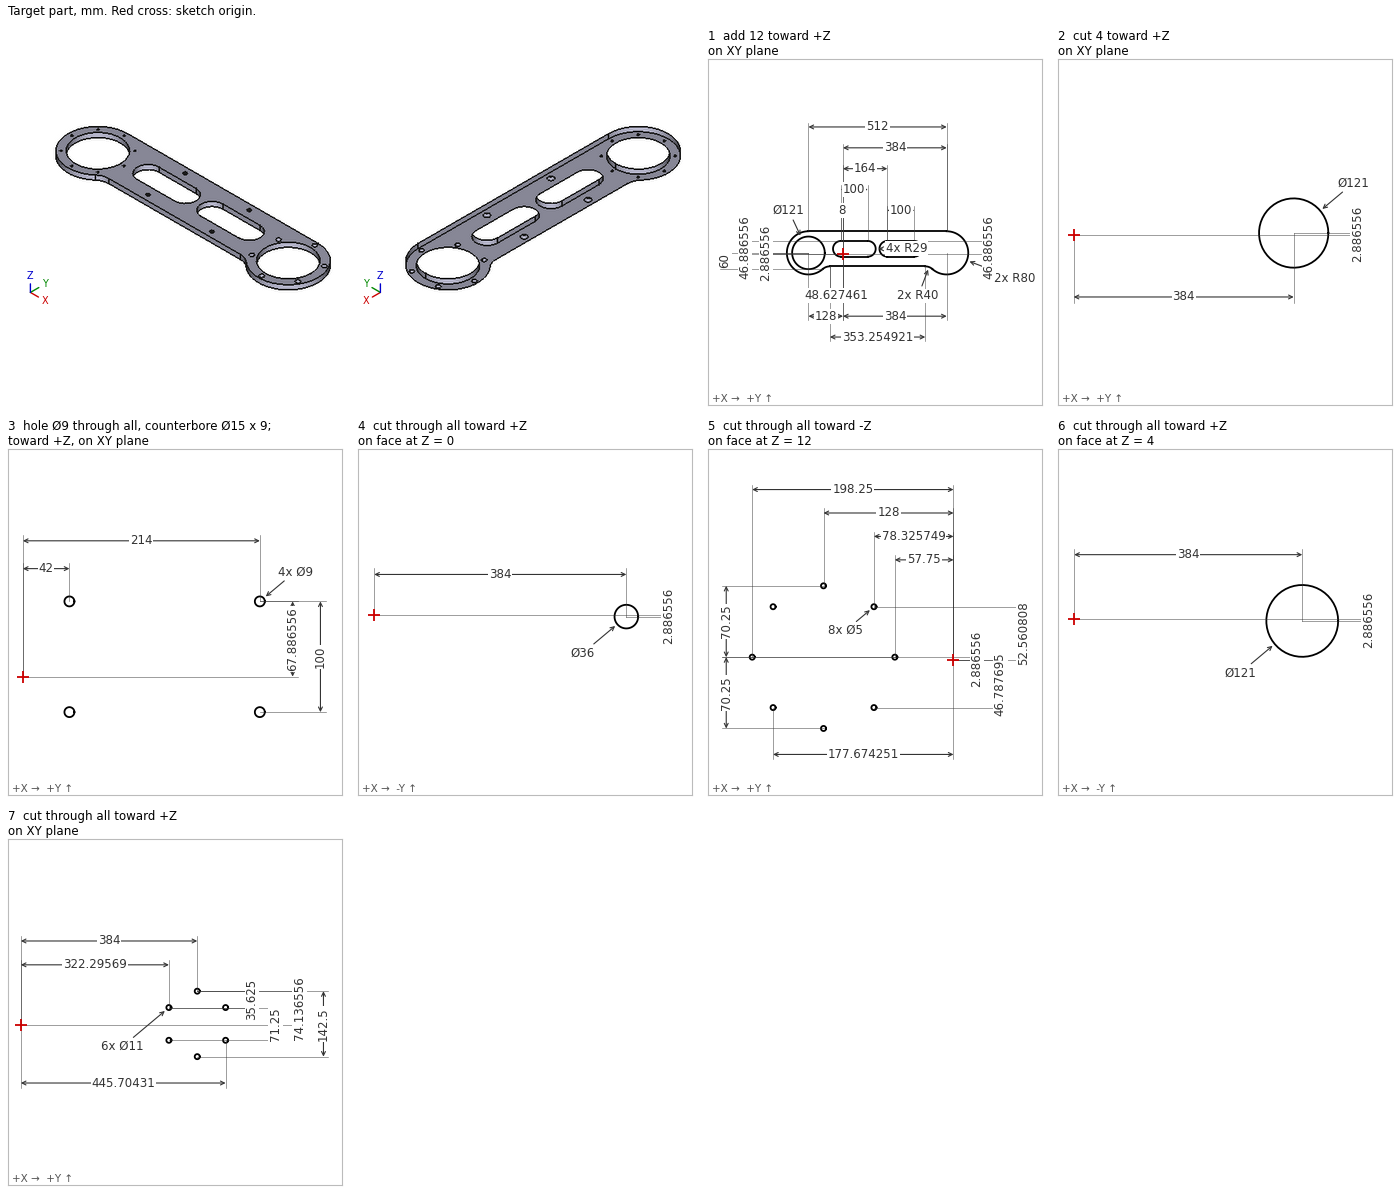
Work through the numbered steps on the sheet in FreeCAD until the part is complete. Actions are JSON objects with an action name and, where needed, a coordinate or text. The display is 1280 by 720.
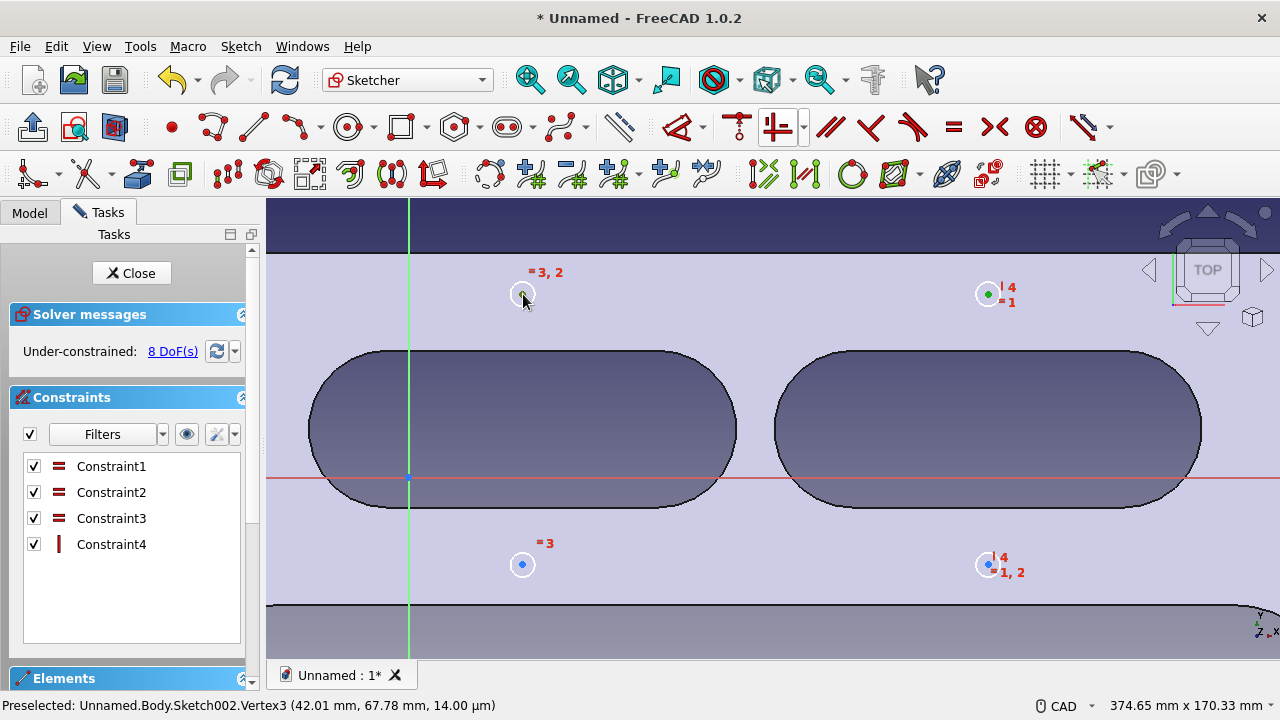
{"action": "left_click", "coordinate": [804, 128]}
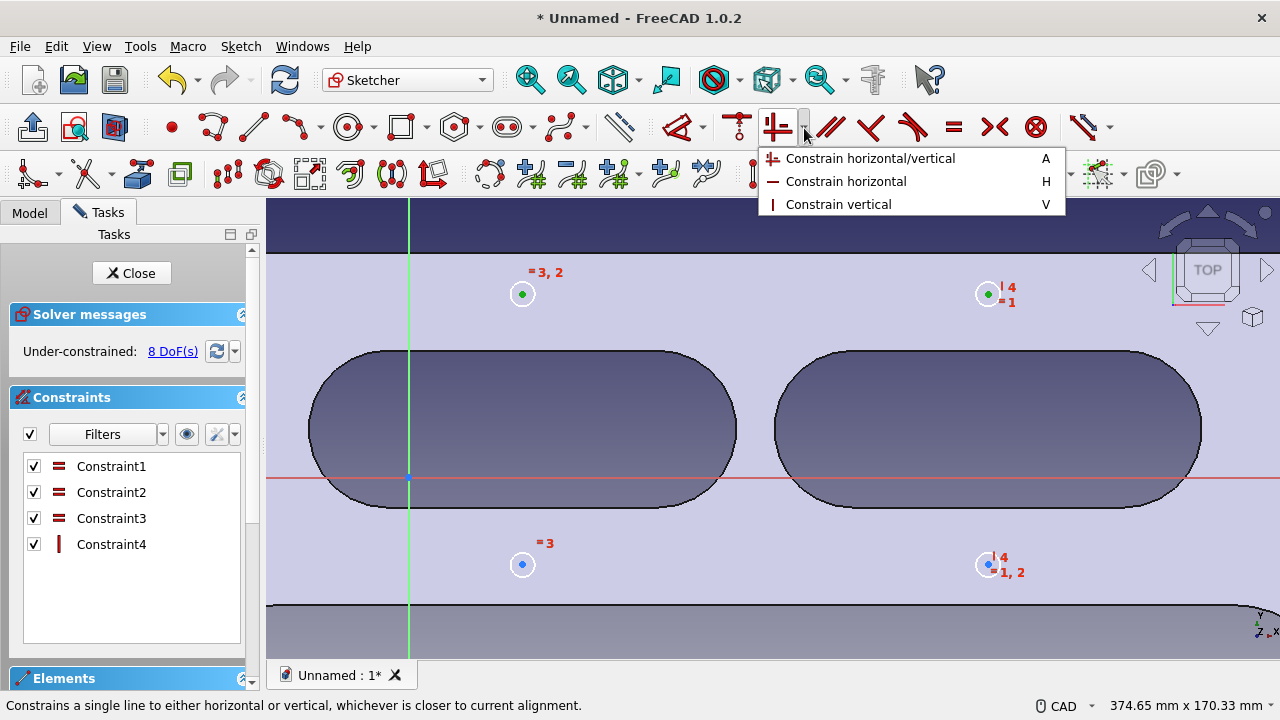
{"action": "left_click", "coordinate": [912, 182]}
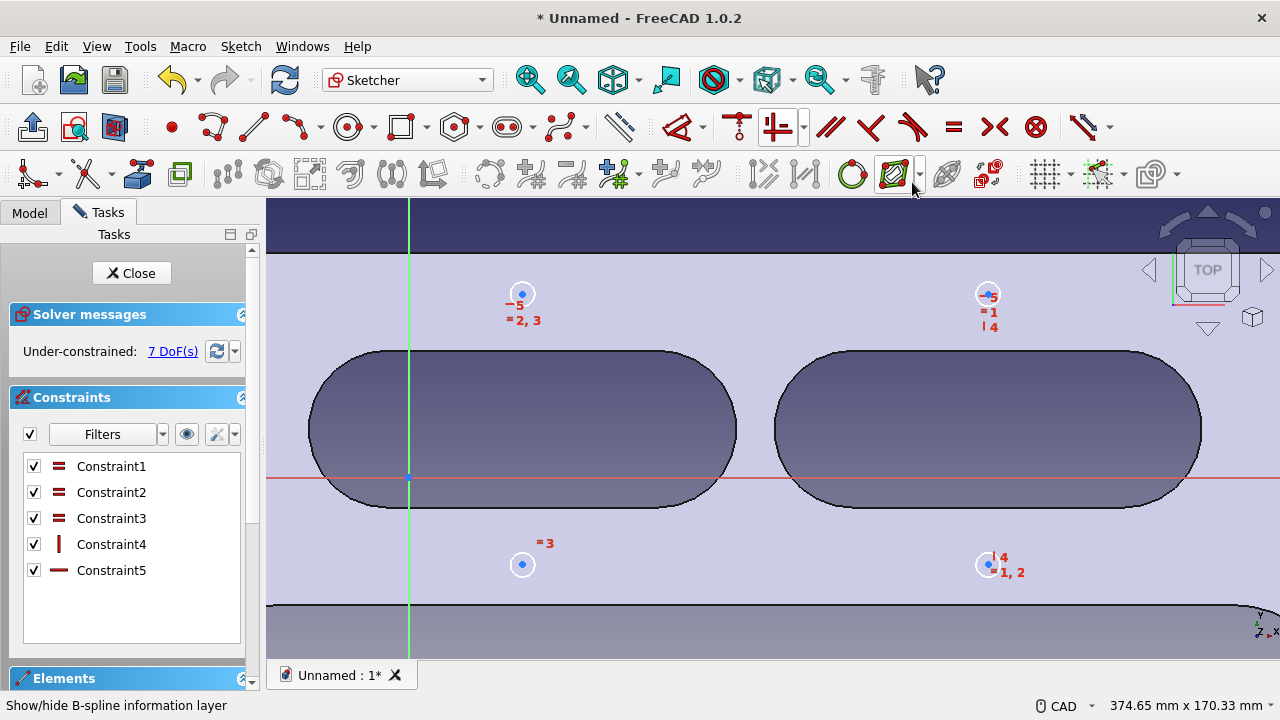
{"action": "left_click", "coordinate": [523, 294]}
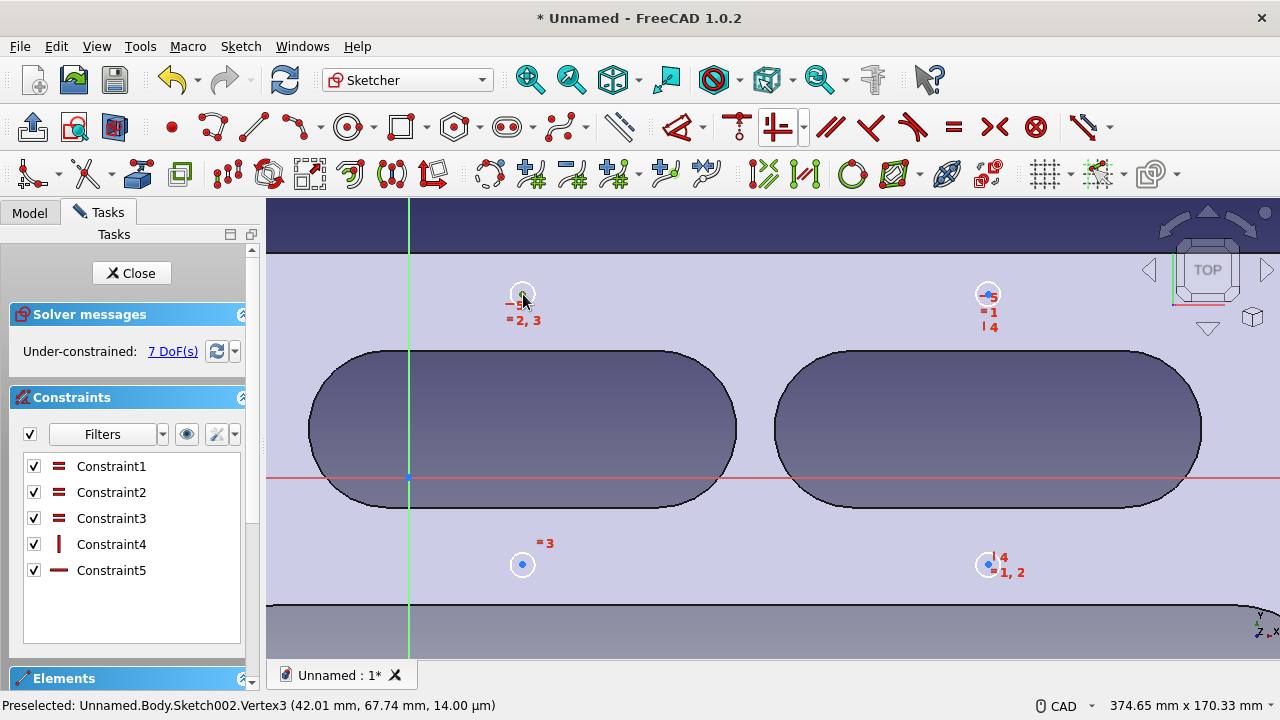
{"action": "left_click", "coordinate": [523, 565]}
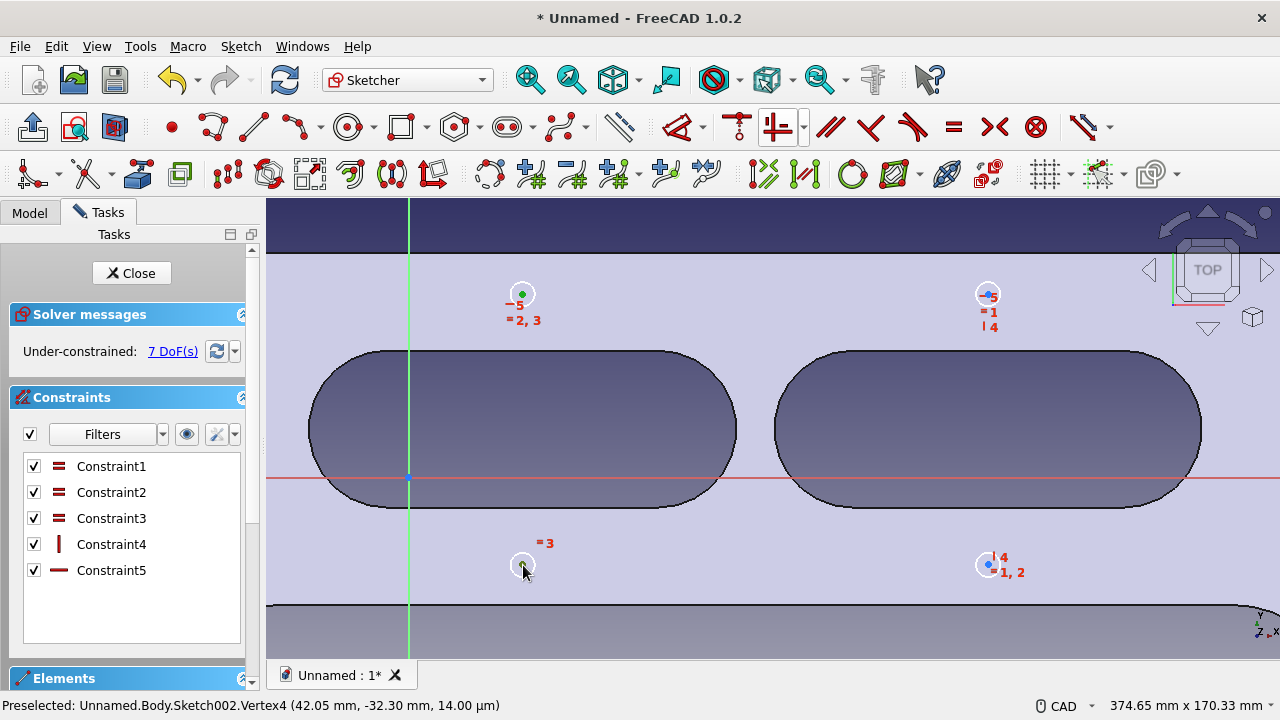
{"action": "left_click", "coordinate": [804, 128]}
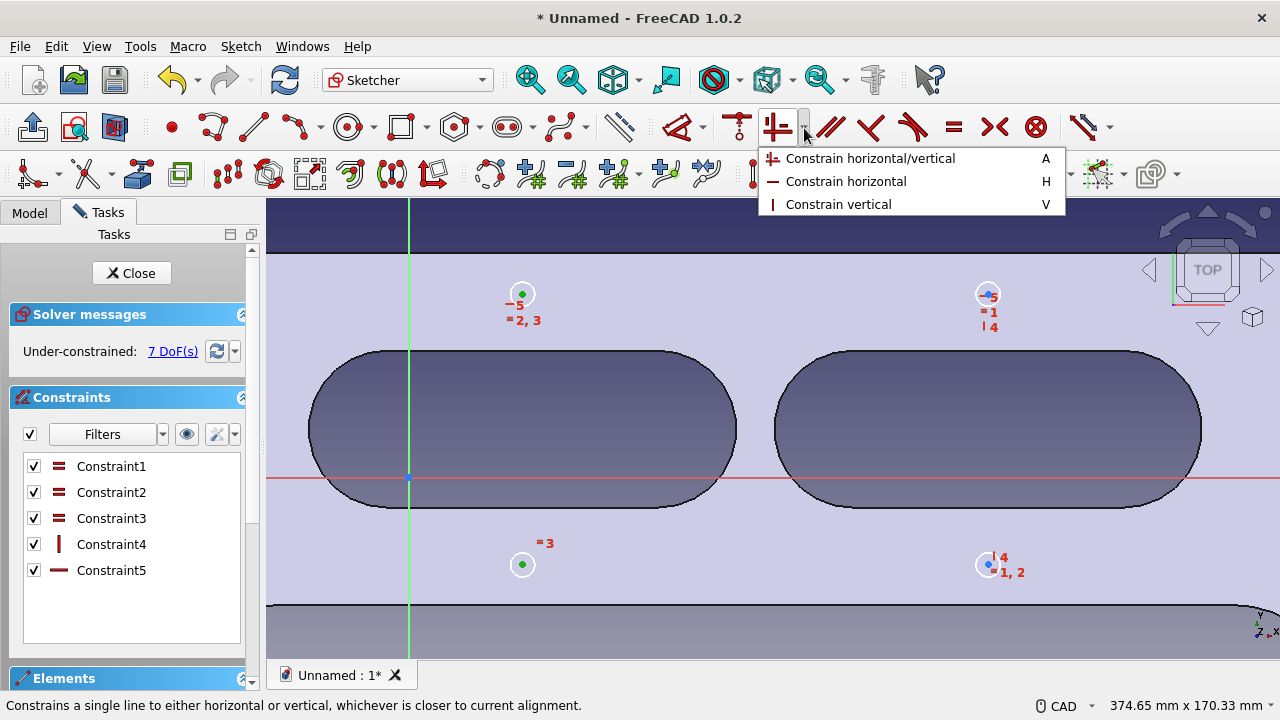
{"action": "left_click", "coordinate": [912, 204]}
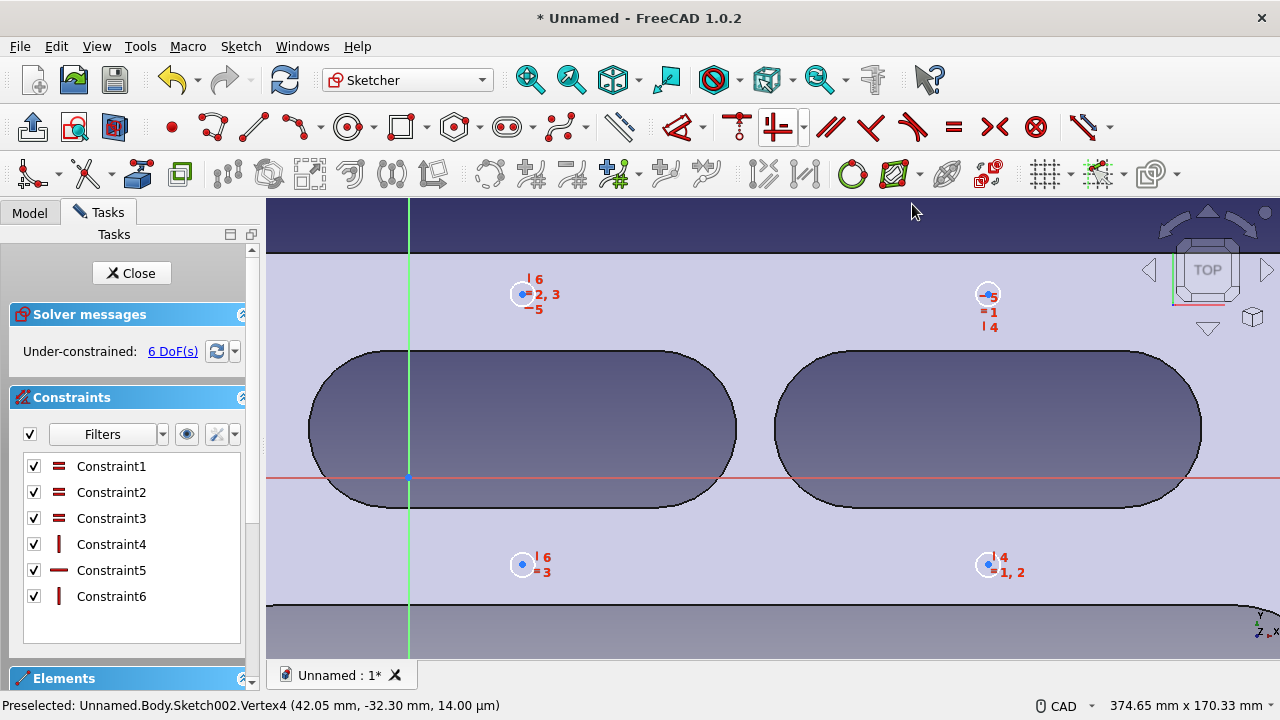
{"action": "left_click", "coordinate": [988, 565]}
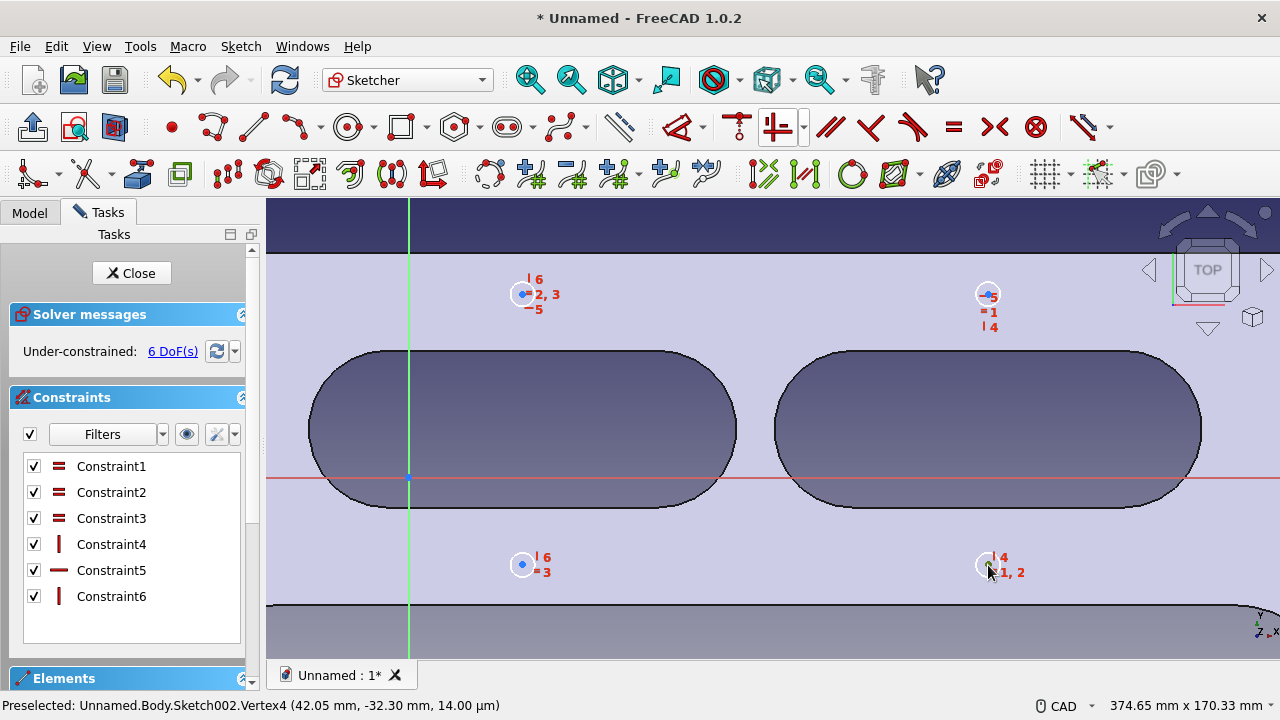
{"action": "left_click", "coordinate": [523, 565]}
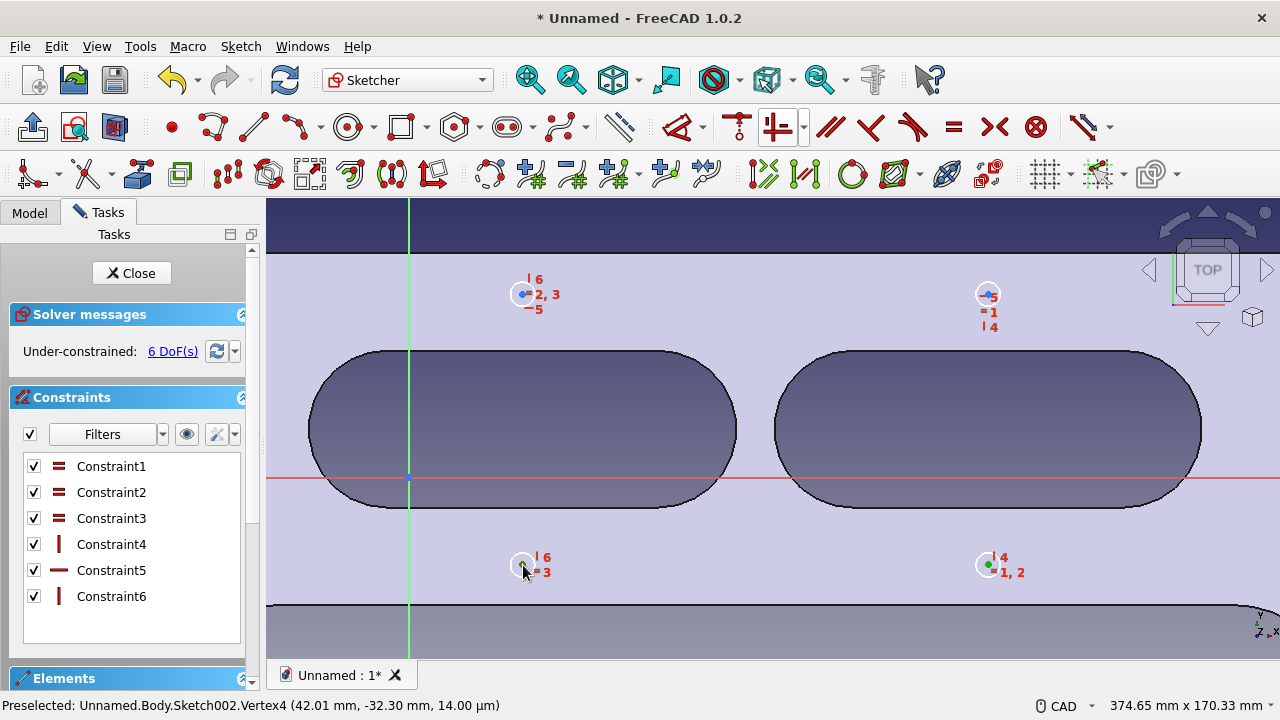
{"action": "left_click", "coordinate": [804, 128]}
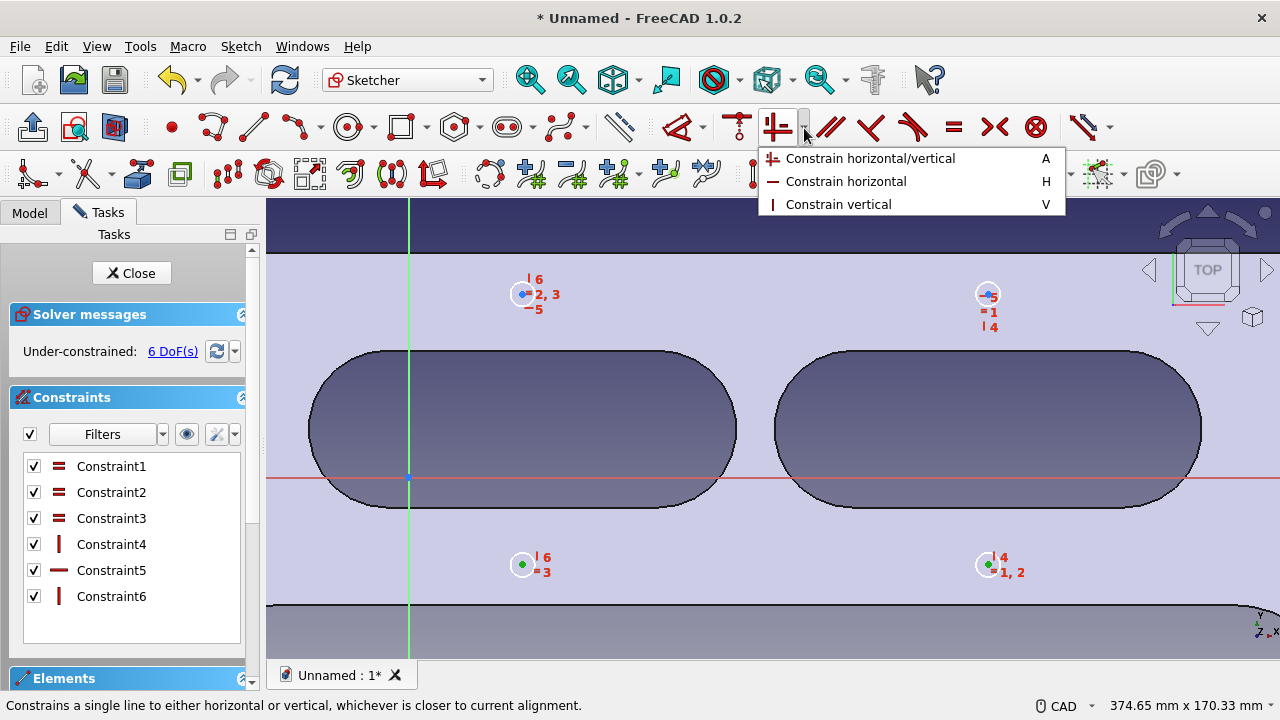
{"action": "left_click", "coordinate": [912, 182]}